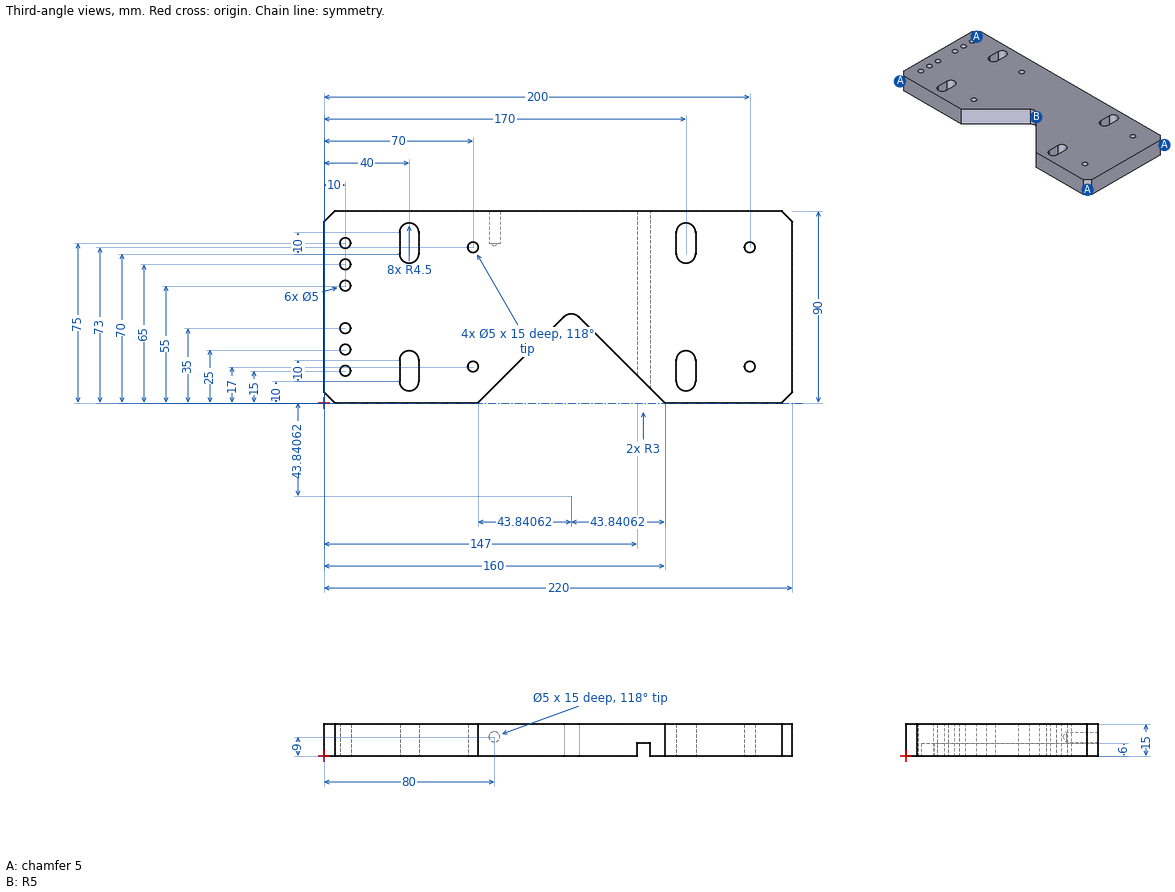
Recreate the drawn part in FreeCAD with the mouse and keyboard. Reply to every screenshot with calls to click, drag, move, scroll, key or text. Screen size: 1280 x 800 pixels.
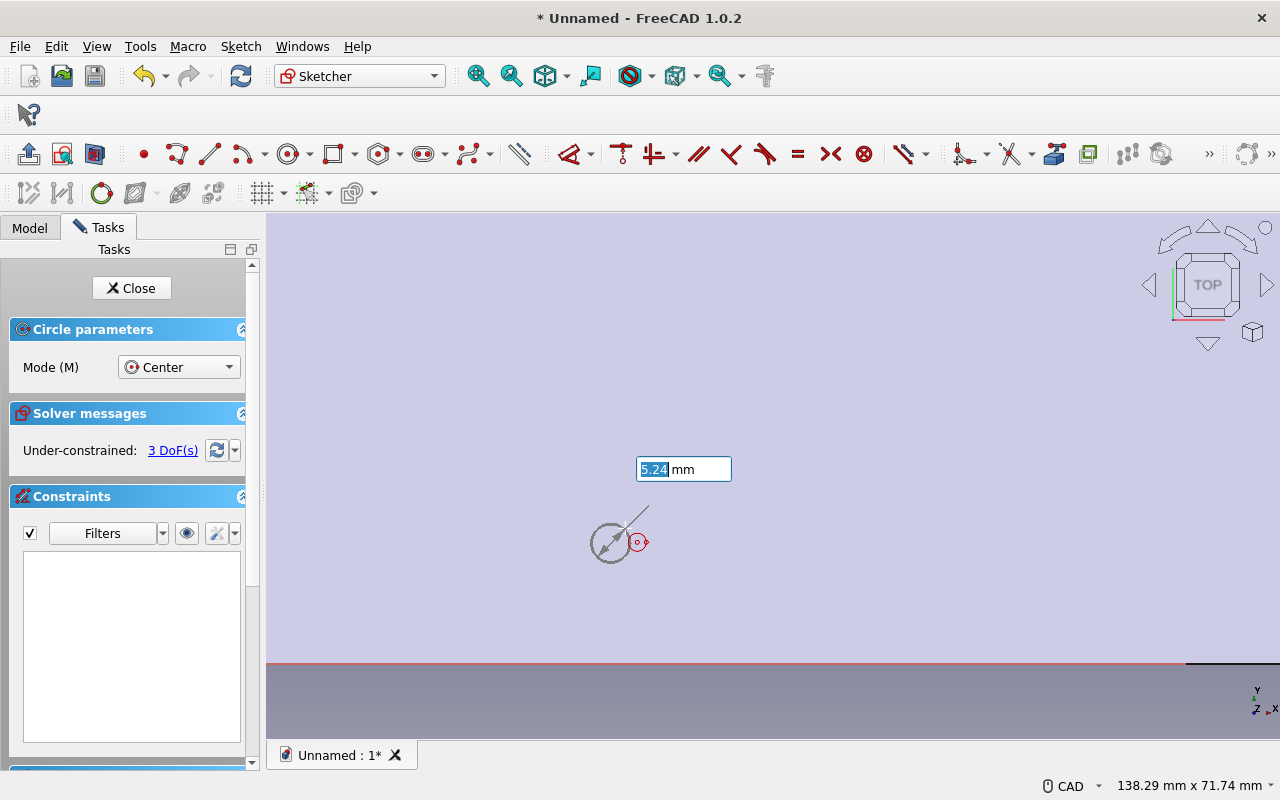
click(625, 527)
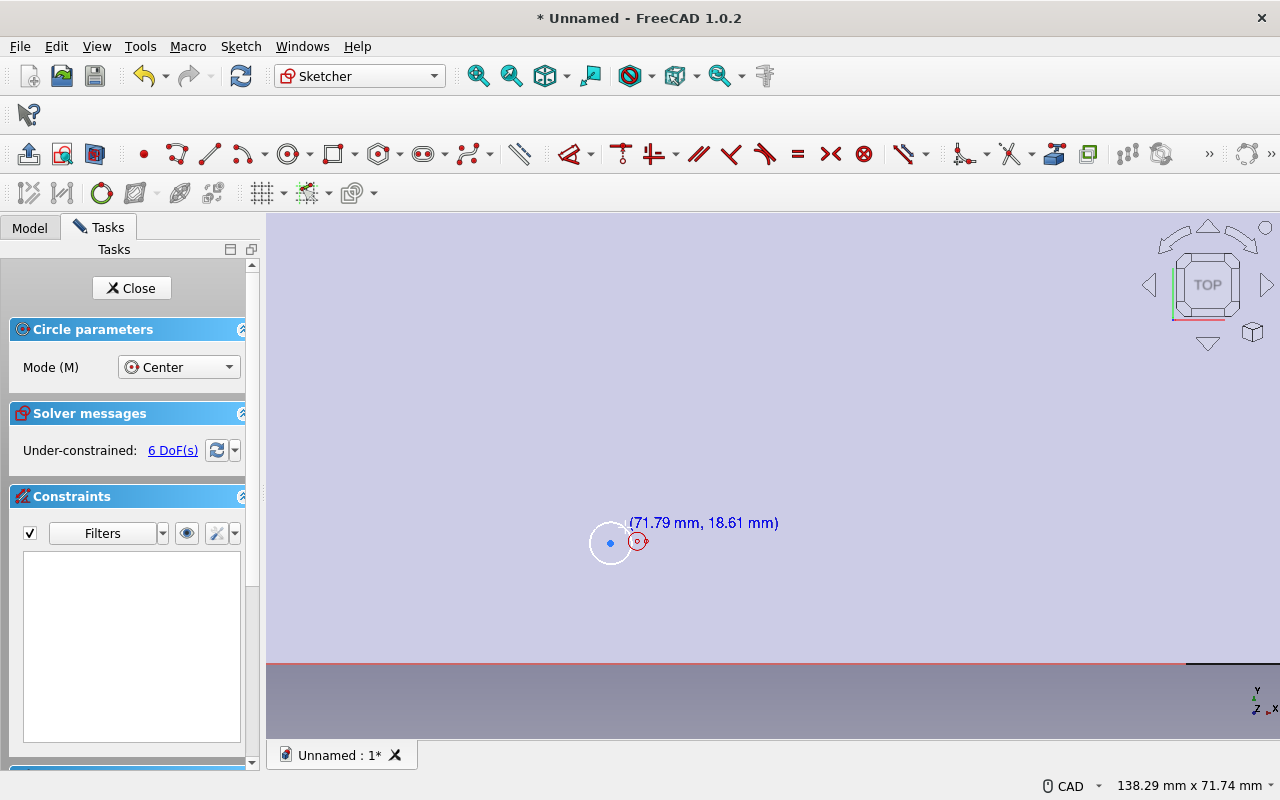
scroll(625, 527, down, 5)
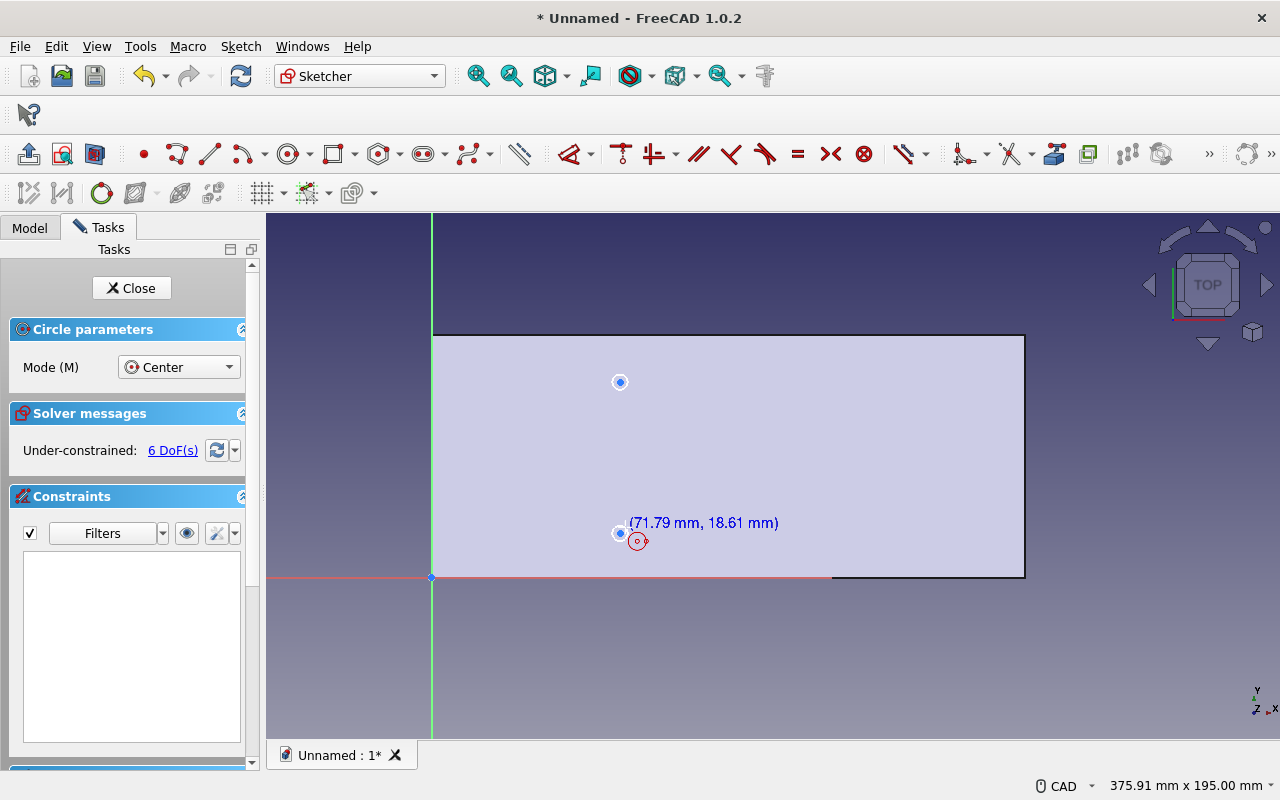
scroll(971, 381, up, 7)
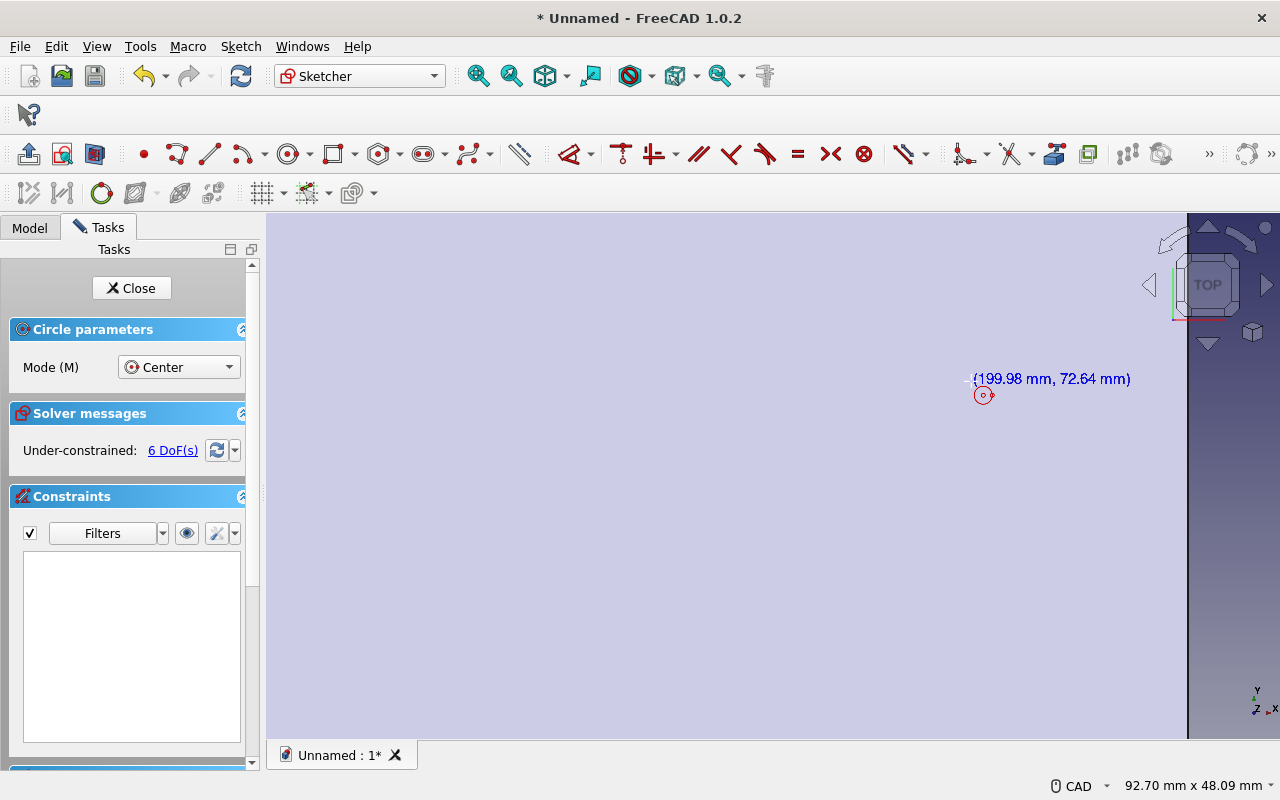
scroll(971, 381, down, 7)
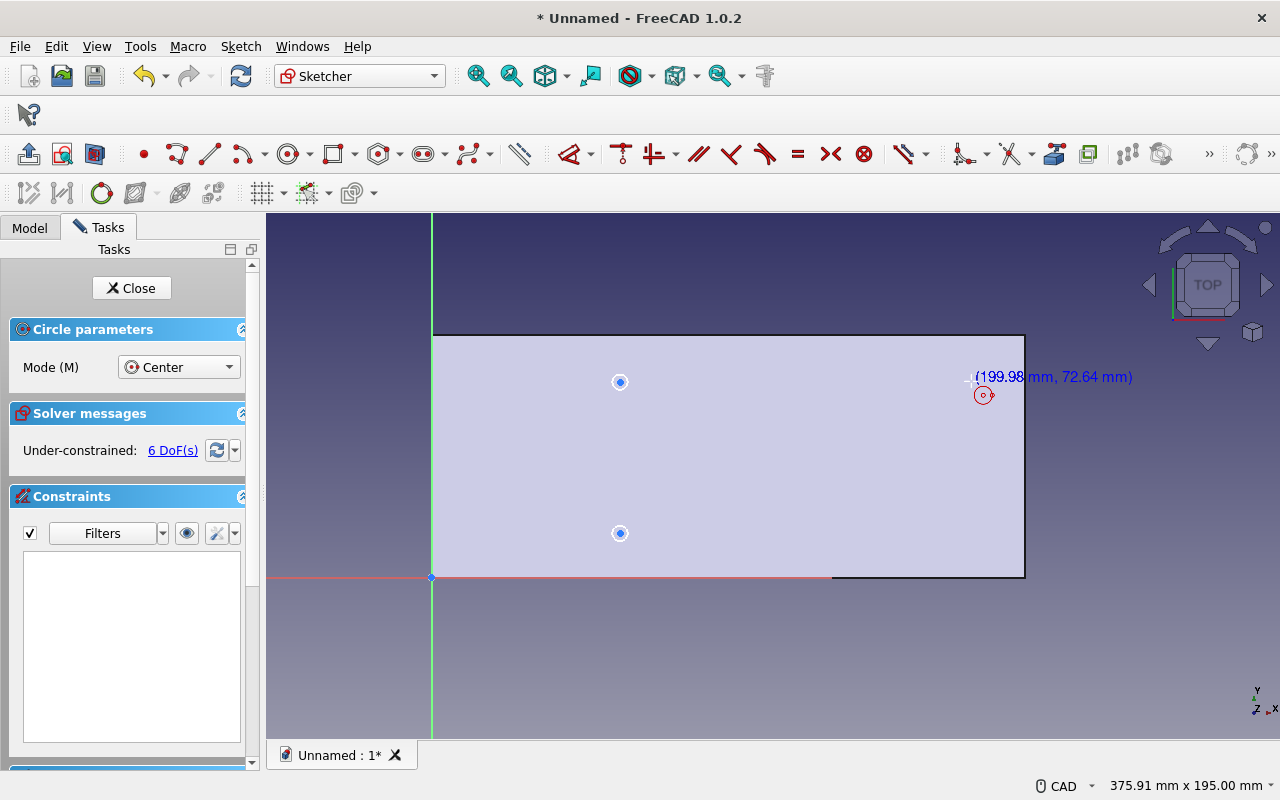
click(971, 381)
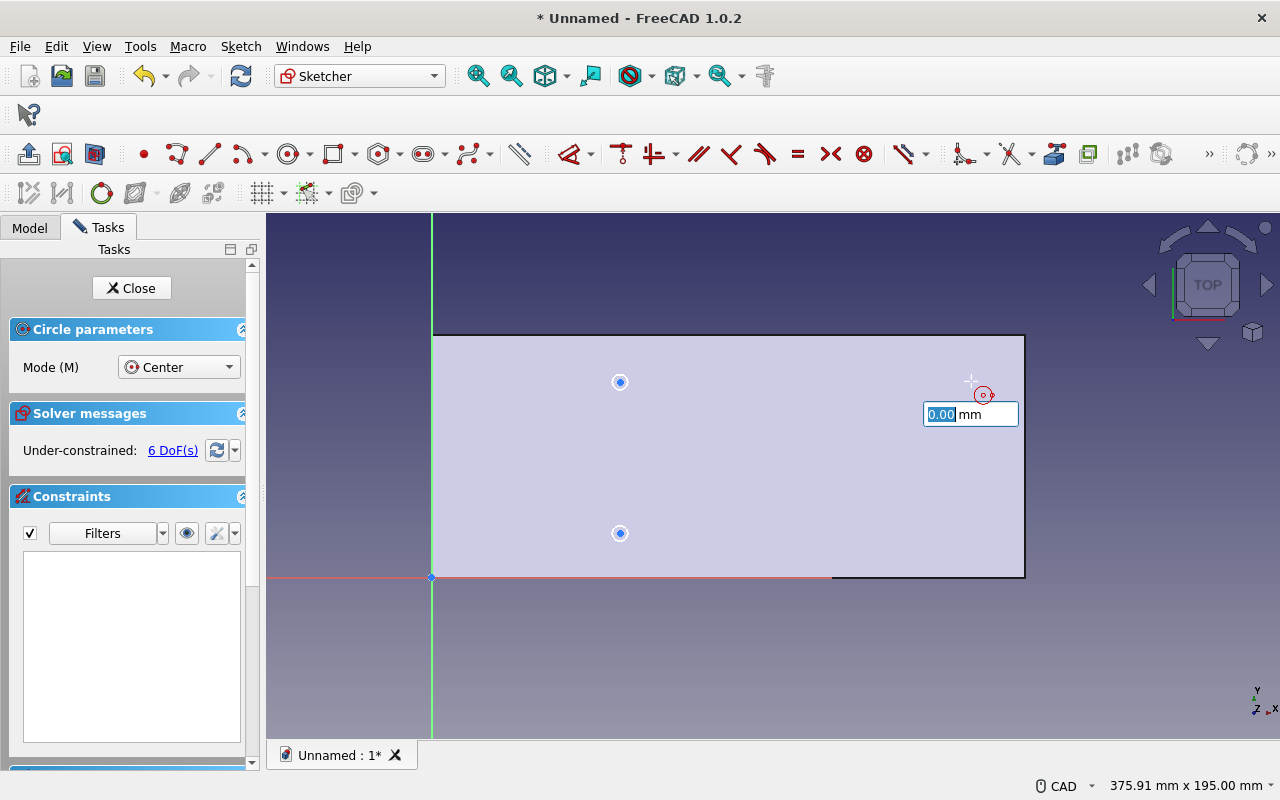
scroll(976, 376, up, 5)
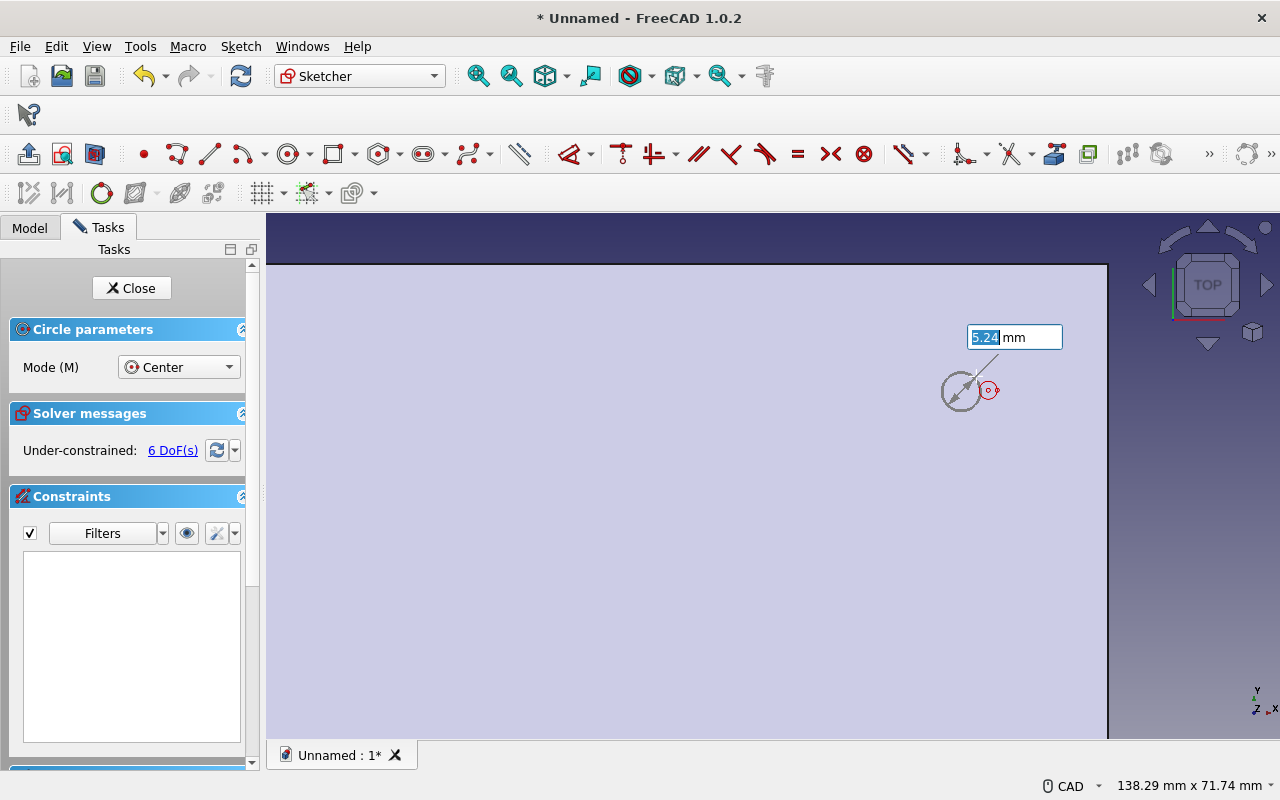
click(974, 376)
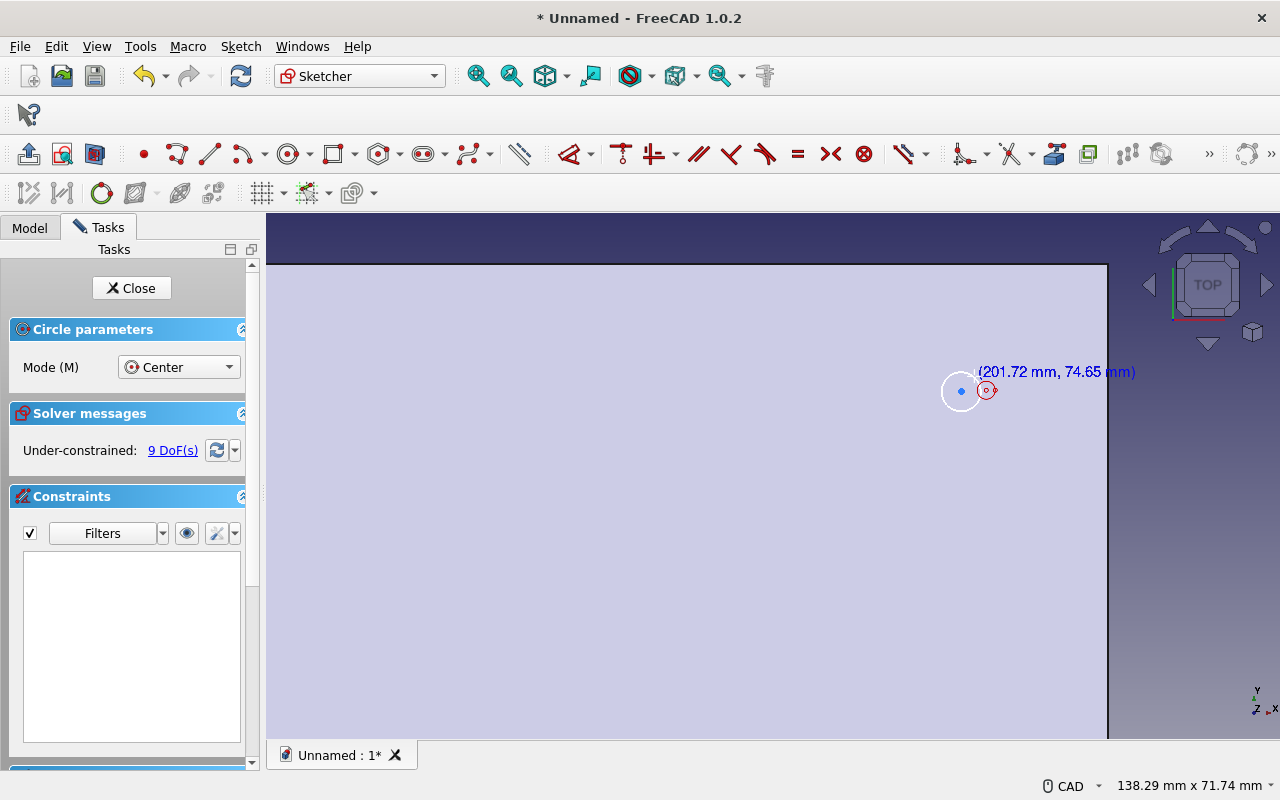
scroll(976, 376, down, 5)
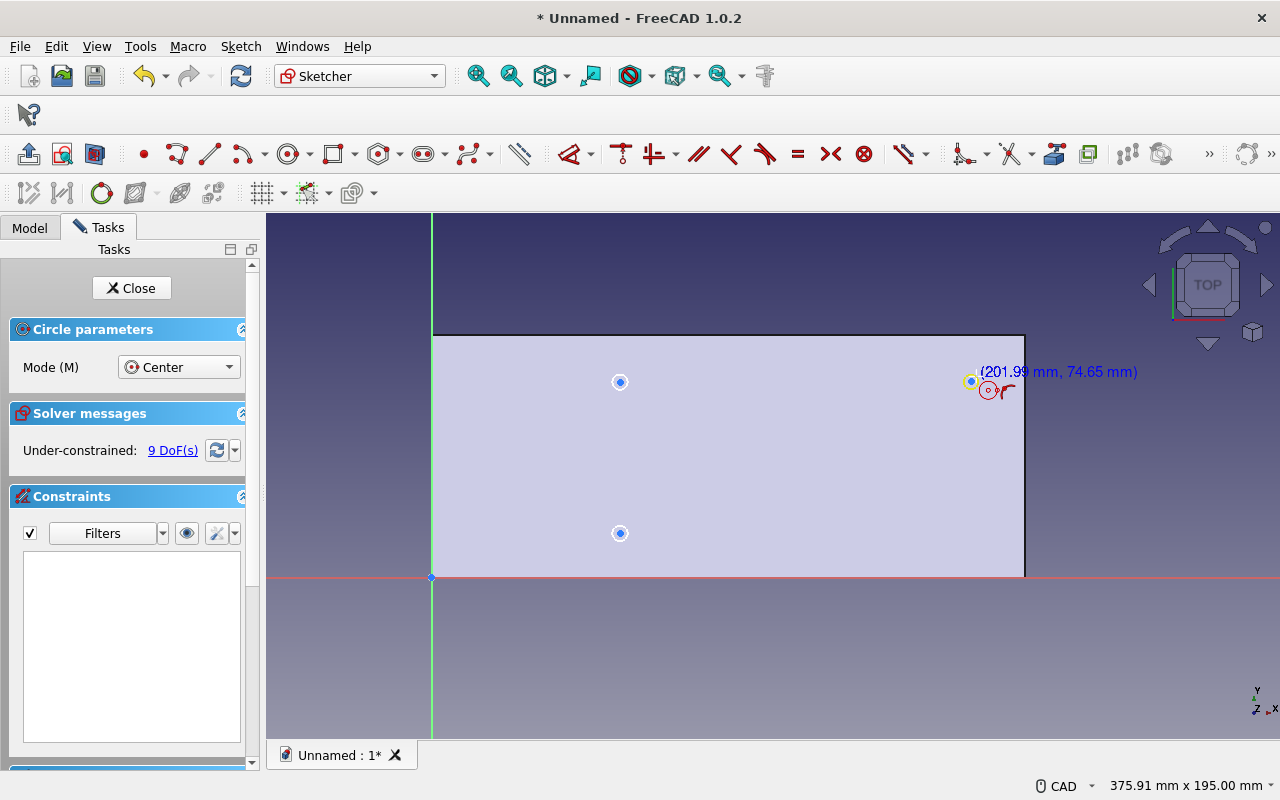
scroll(971, 532, up, 7)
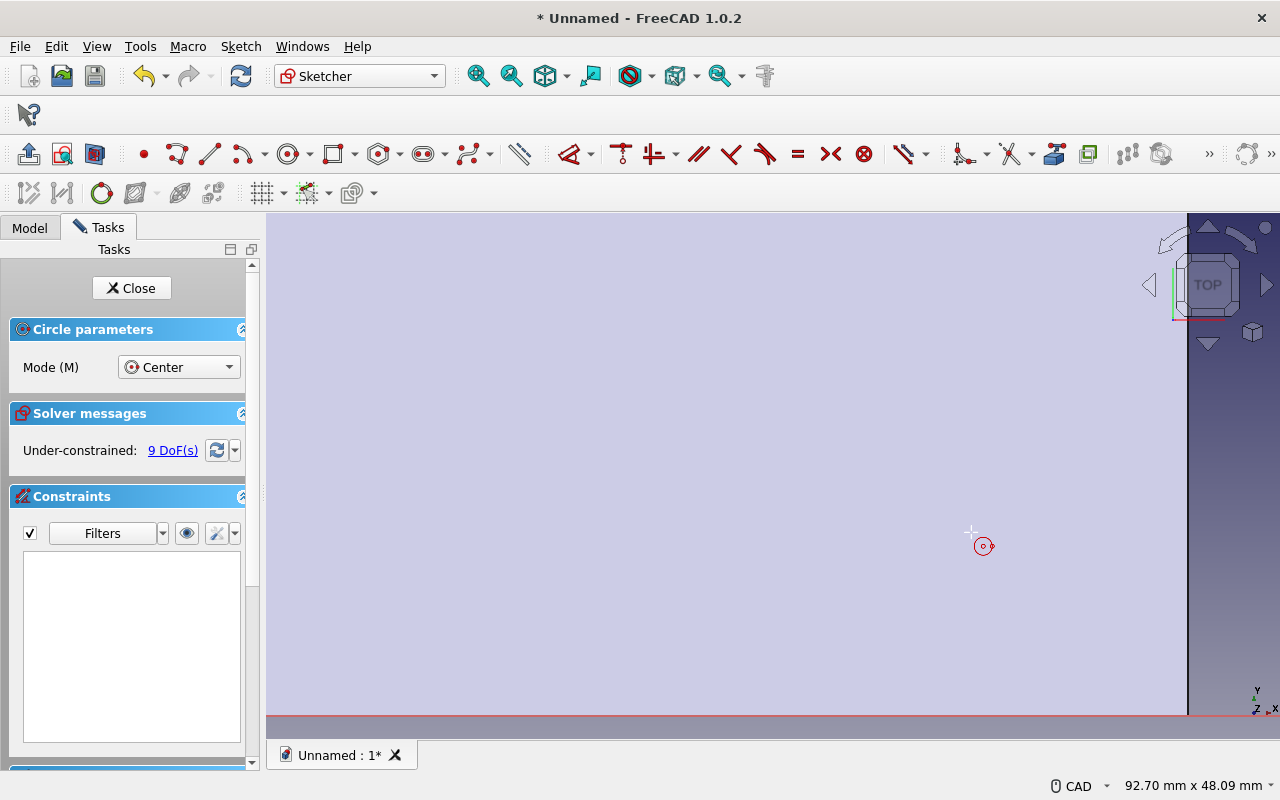
scroll(971, 532, down, 7)